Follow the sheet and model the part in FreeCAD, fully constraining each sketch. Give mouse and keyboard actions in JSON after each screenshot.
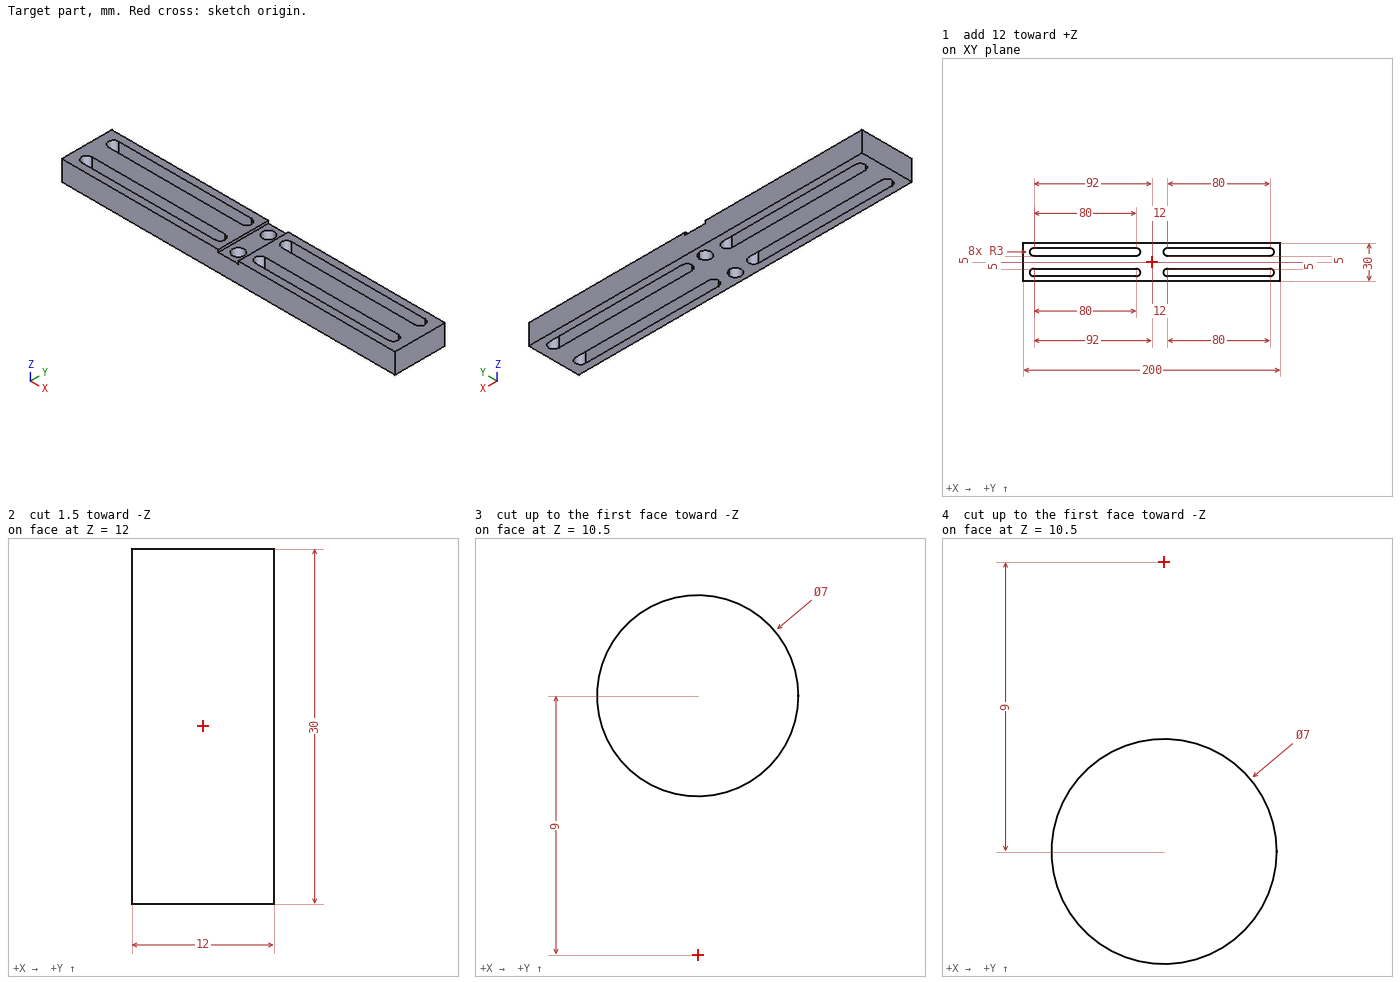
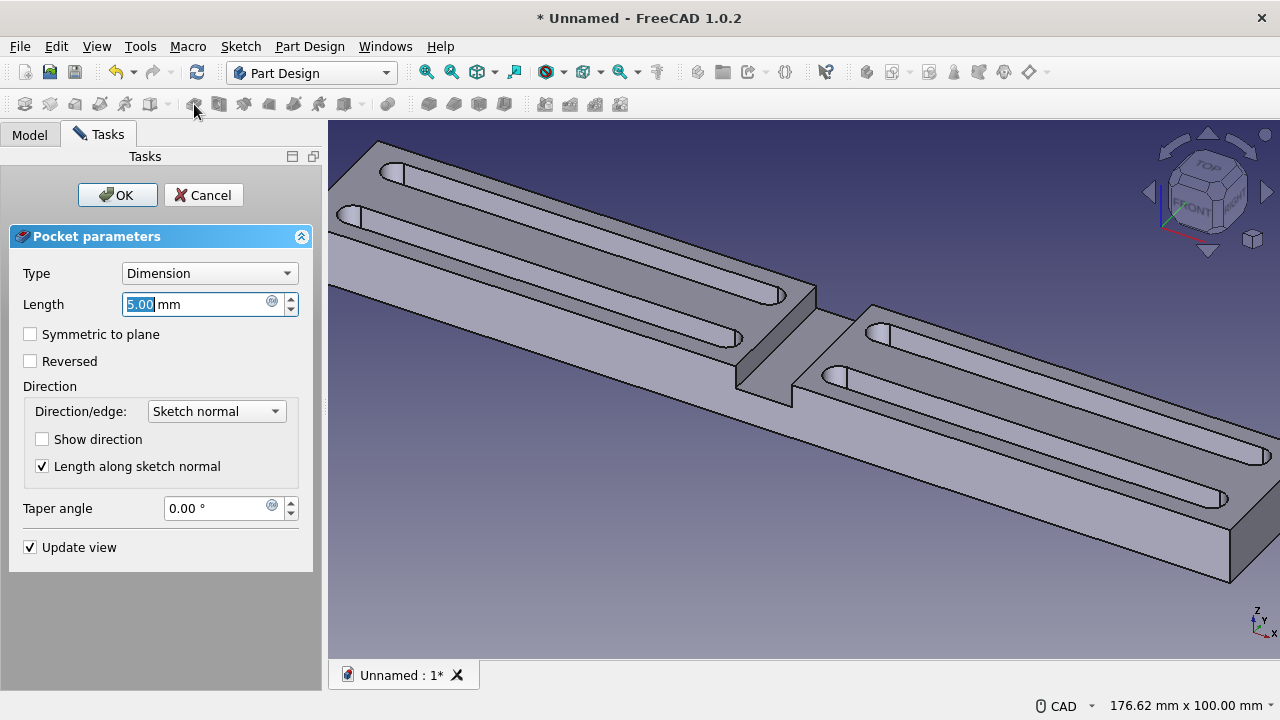
{"action": "type", "text": "1.5"}
{"action": "key", "text": "Tab"}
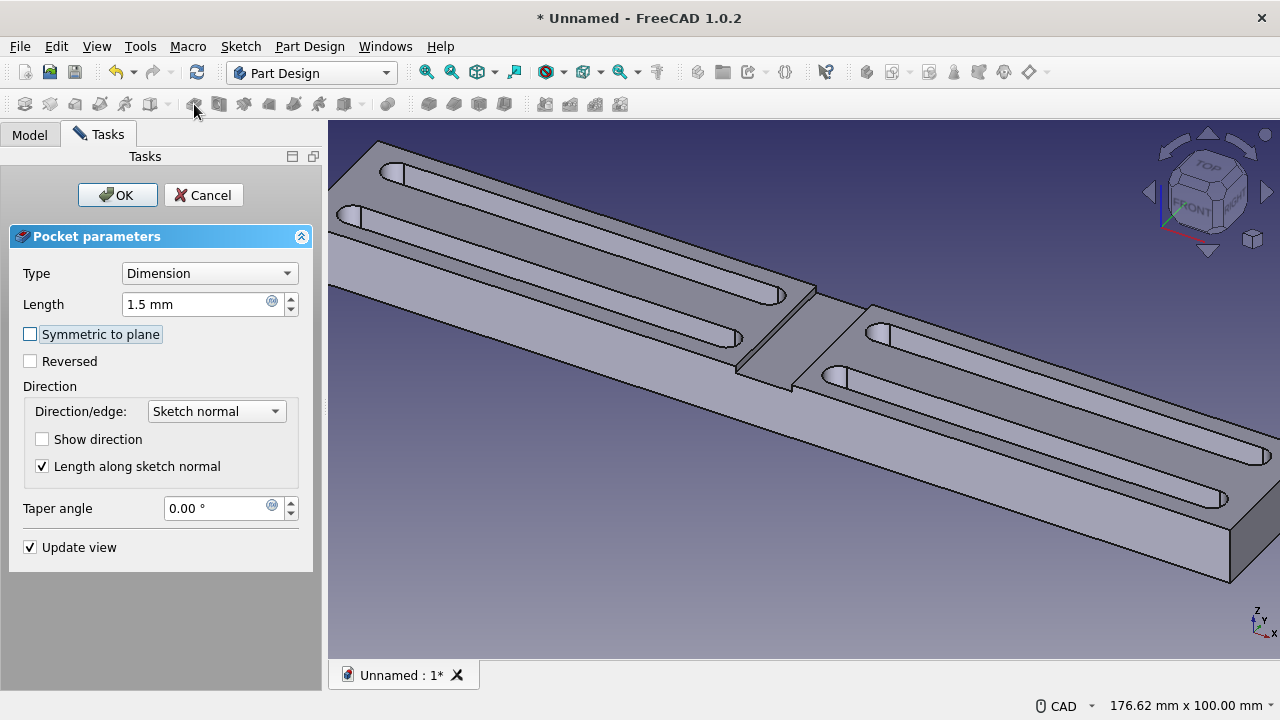
{"action": "left_click", "coordinate": [118, 195]}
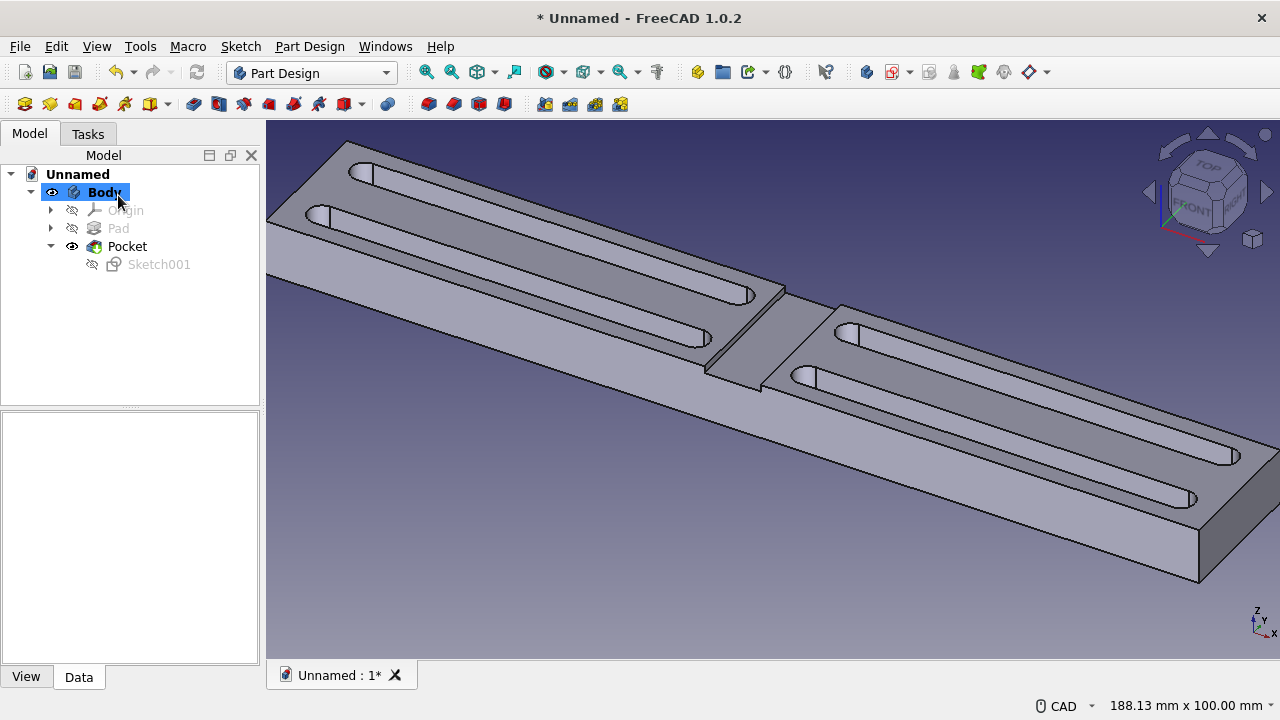
{"action": "left_click", "coordinate": [796, 318]}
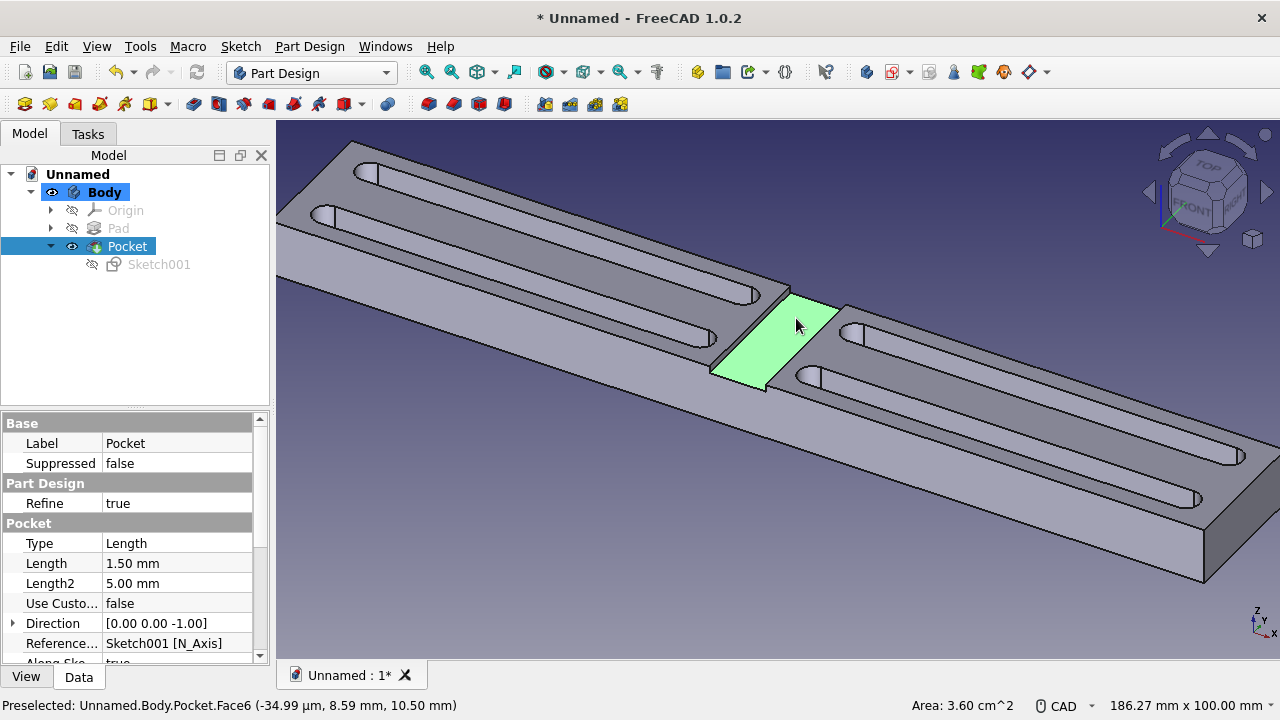
{"action": "left_click", "coordinate": [892, 72]}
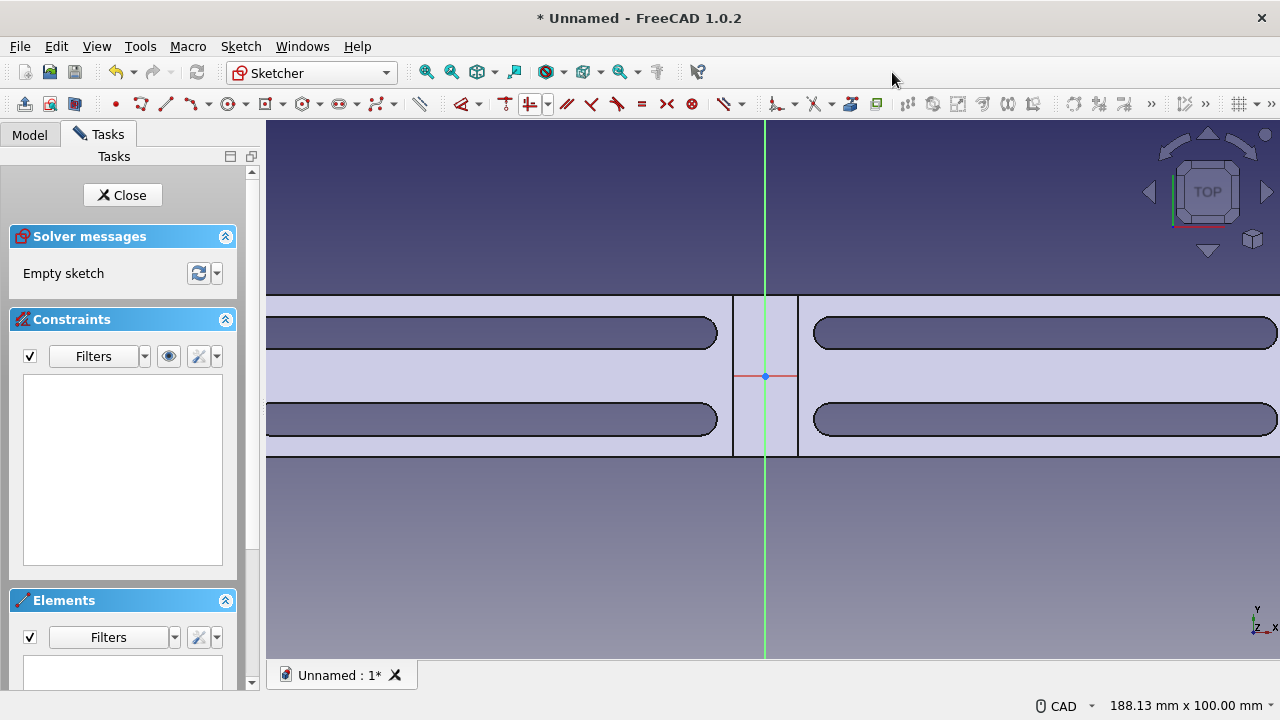
{"action": "scroll", "coordinate": [781, 331], "scroll_direction": "up", "scroll_amount": 8}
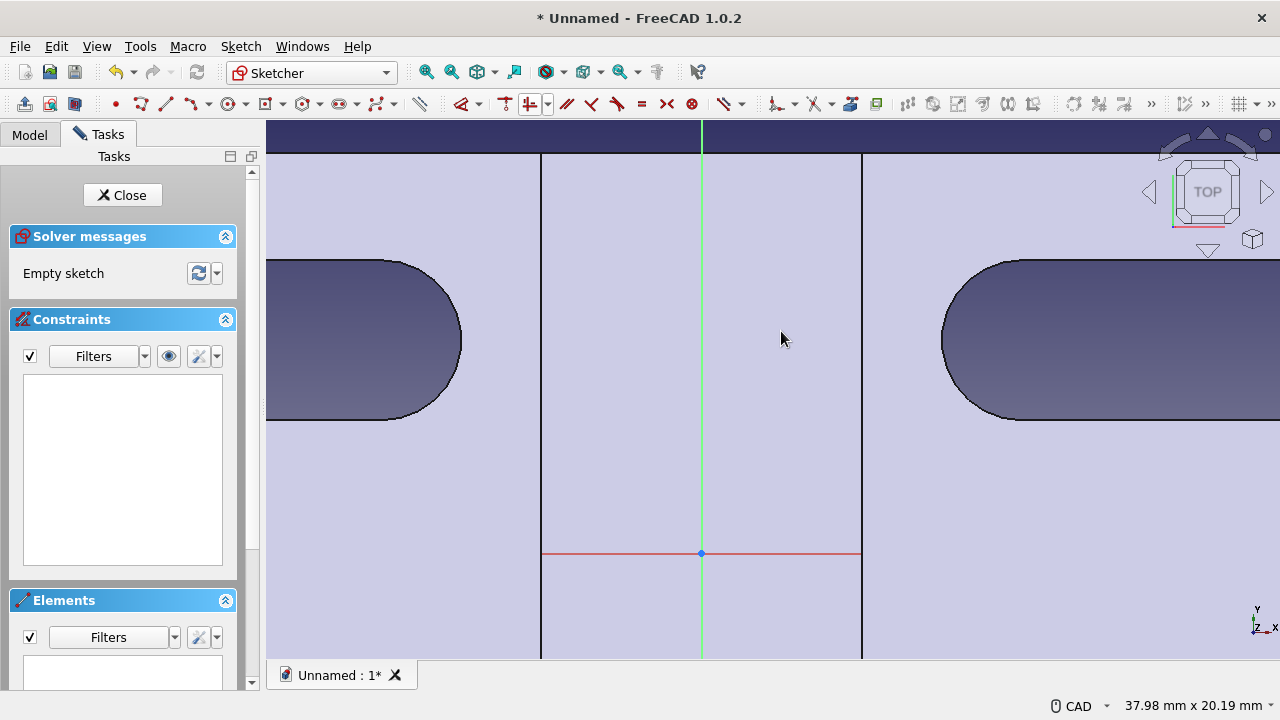
{"action": "left_click", "coordinate": [228, 104]}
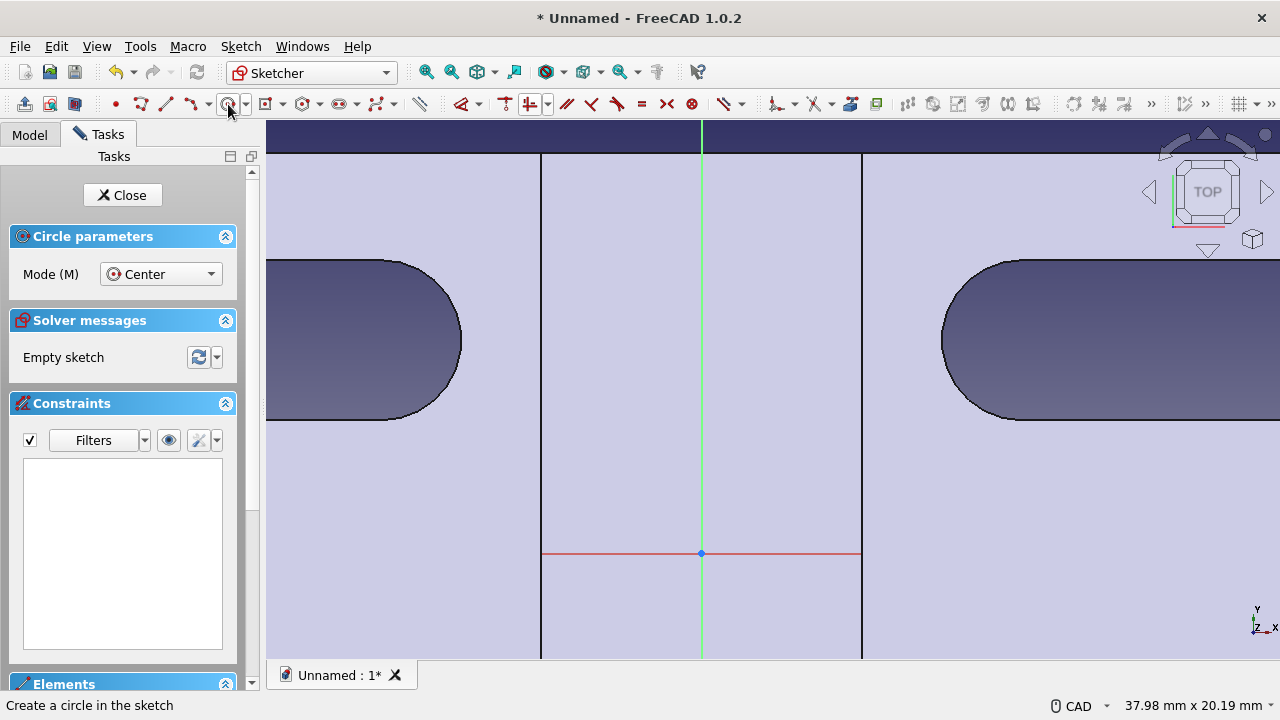
{"action": "left_click", "coordinate": [702, 314]}
{"action": "mouse_move", "coordinate": [768, 247]}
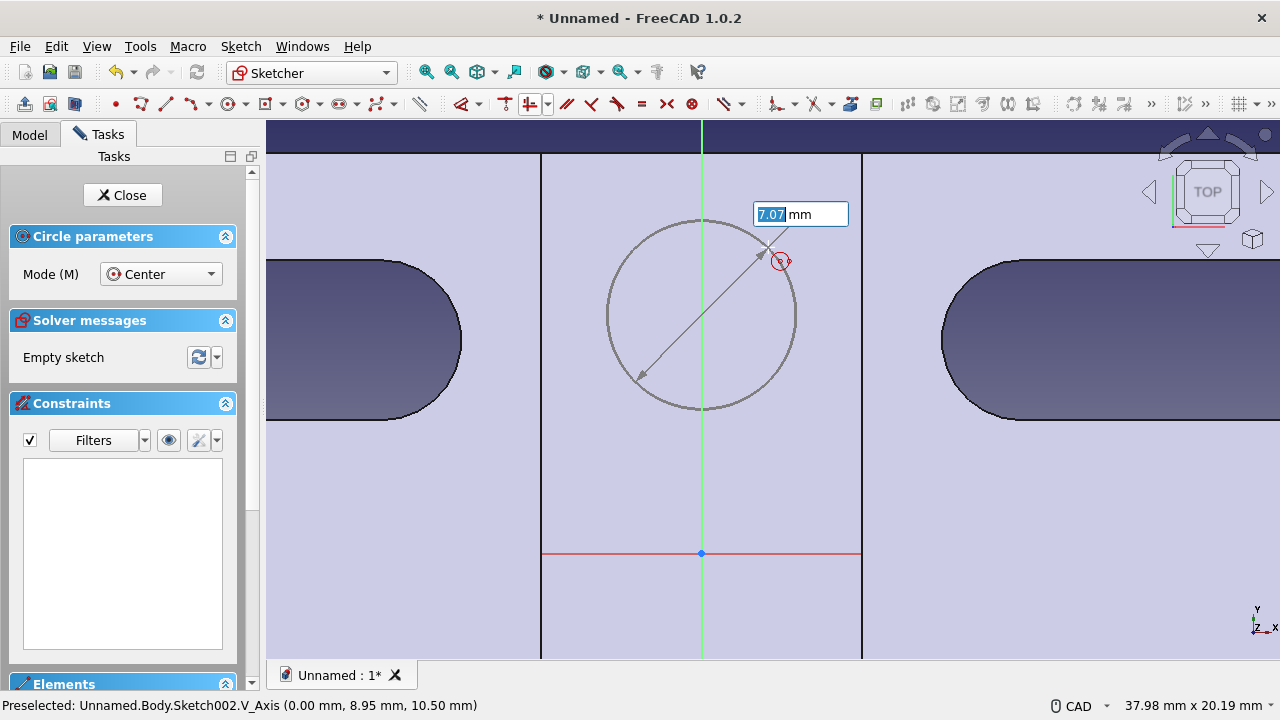
{"action": "type", "text": "7"}
{"action": "key", "text": "Return"}
{"action": "key", "text": "Escape"}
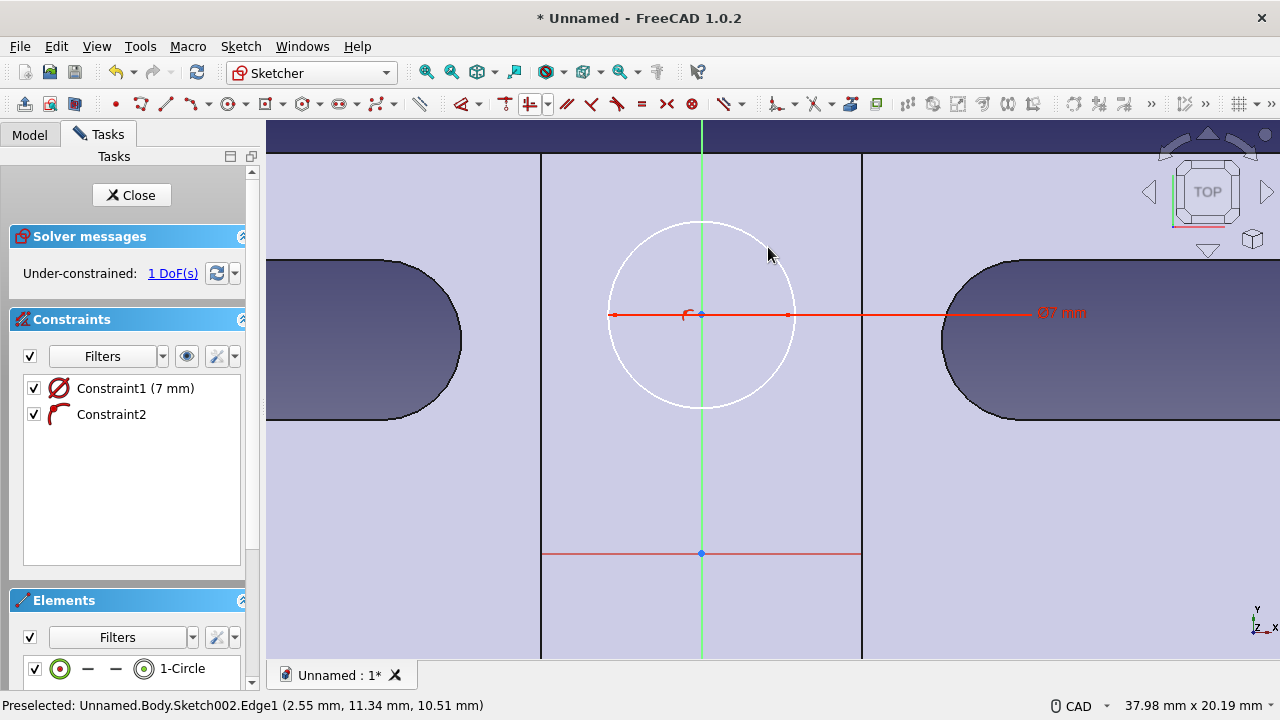
{"action": "left_click", "coordinate": [460, 104]}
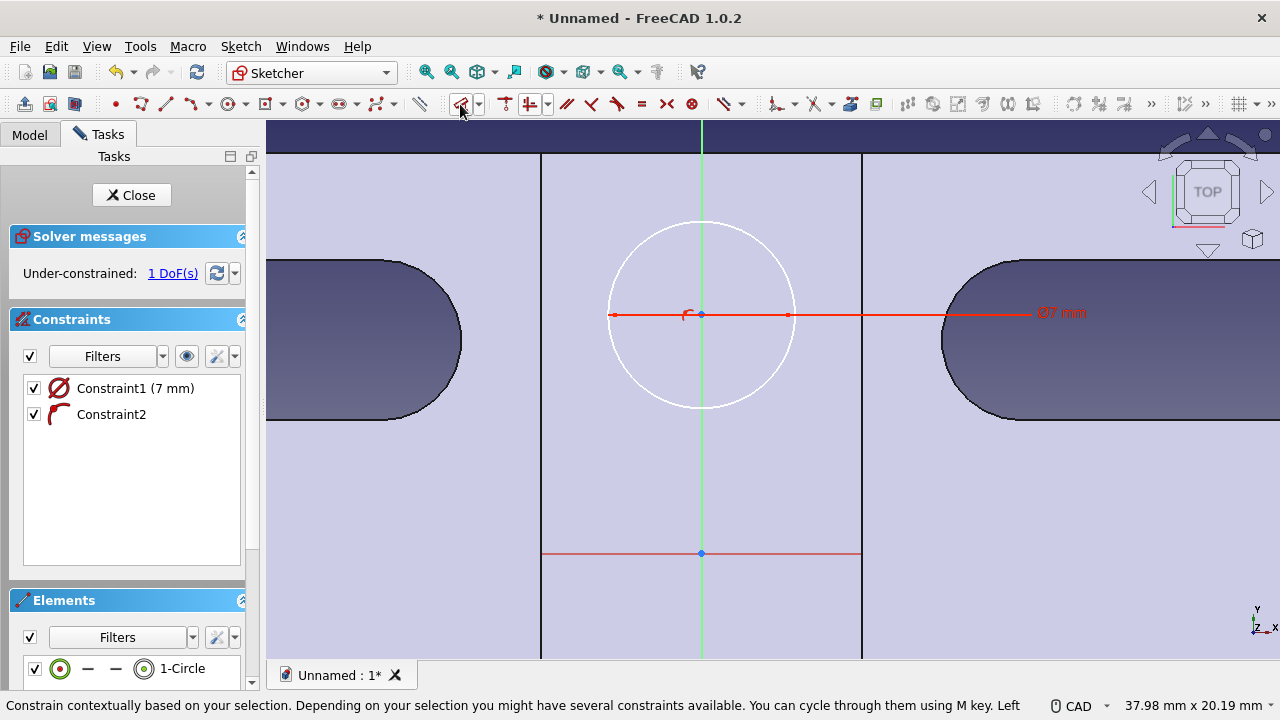
{"action": "left_click", "coordinate": [702, 315]}
{"action": "left_click", "coordinate": [736, 434]}